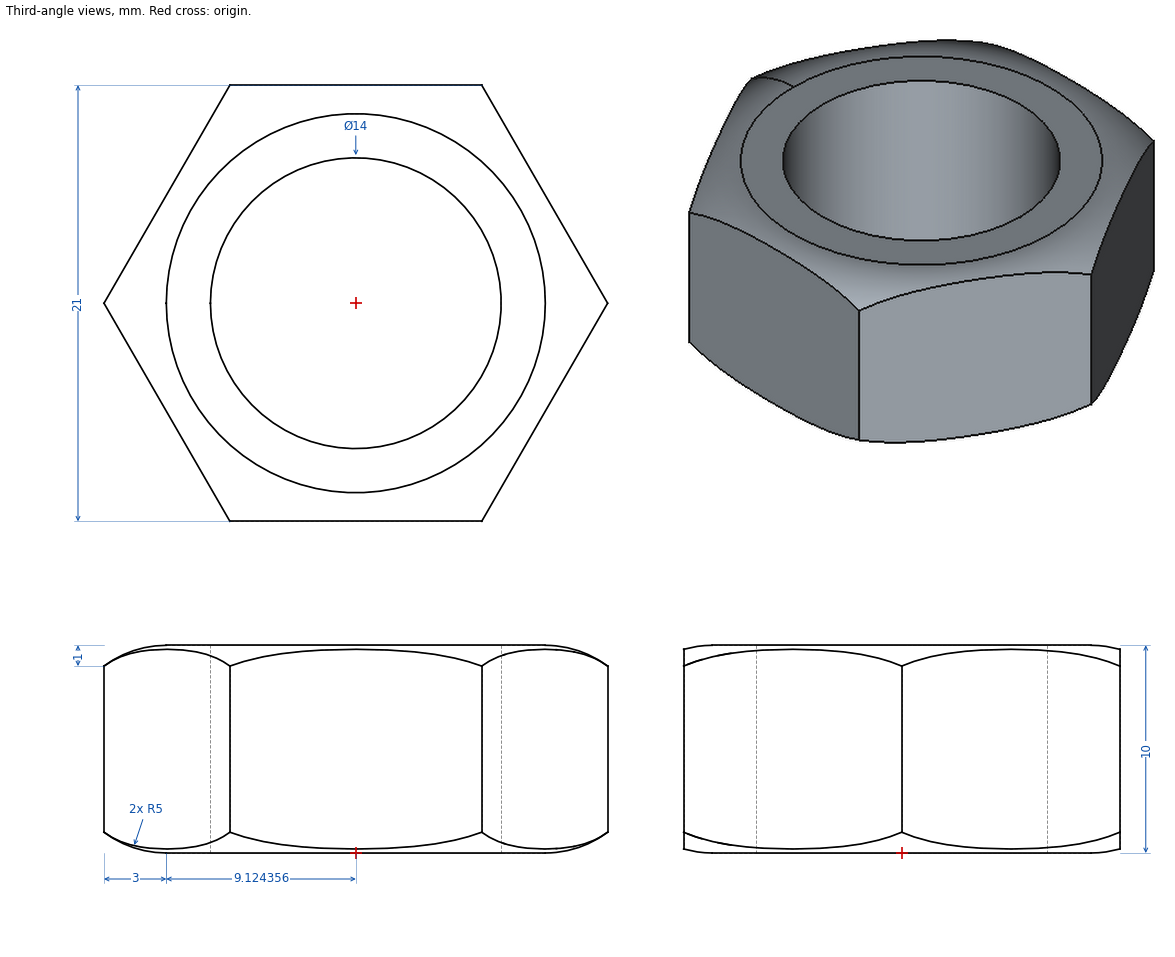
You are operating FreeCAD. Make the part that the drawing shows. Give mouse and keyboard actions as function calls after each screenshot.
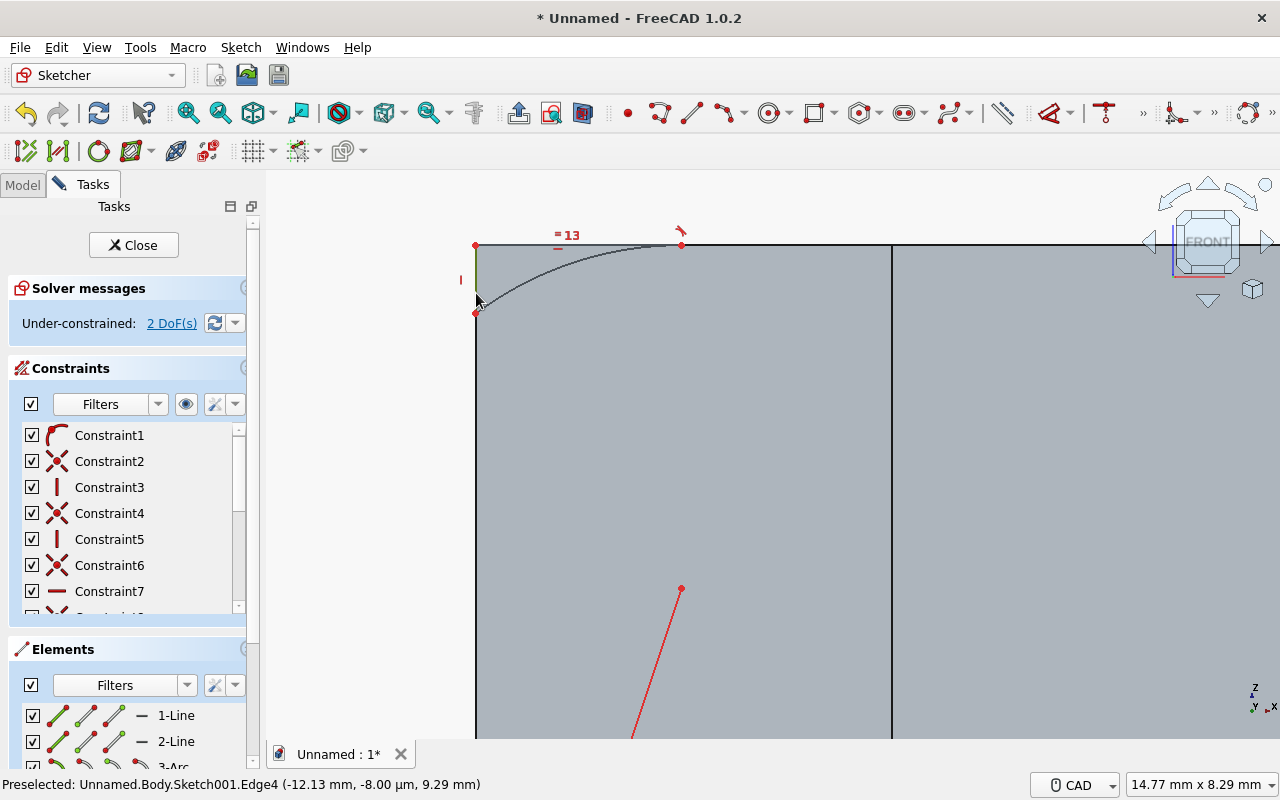
key(i)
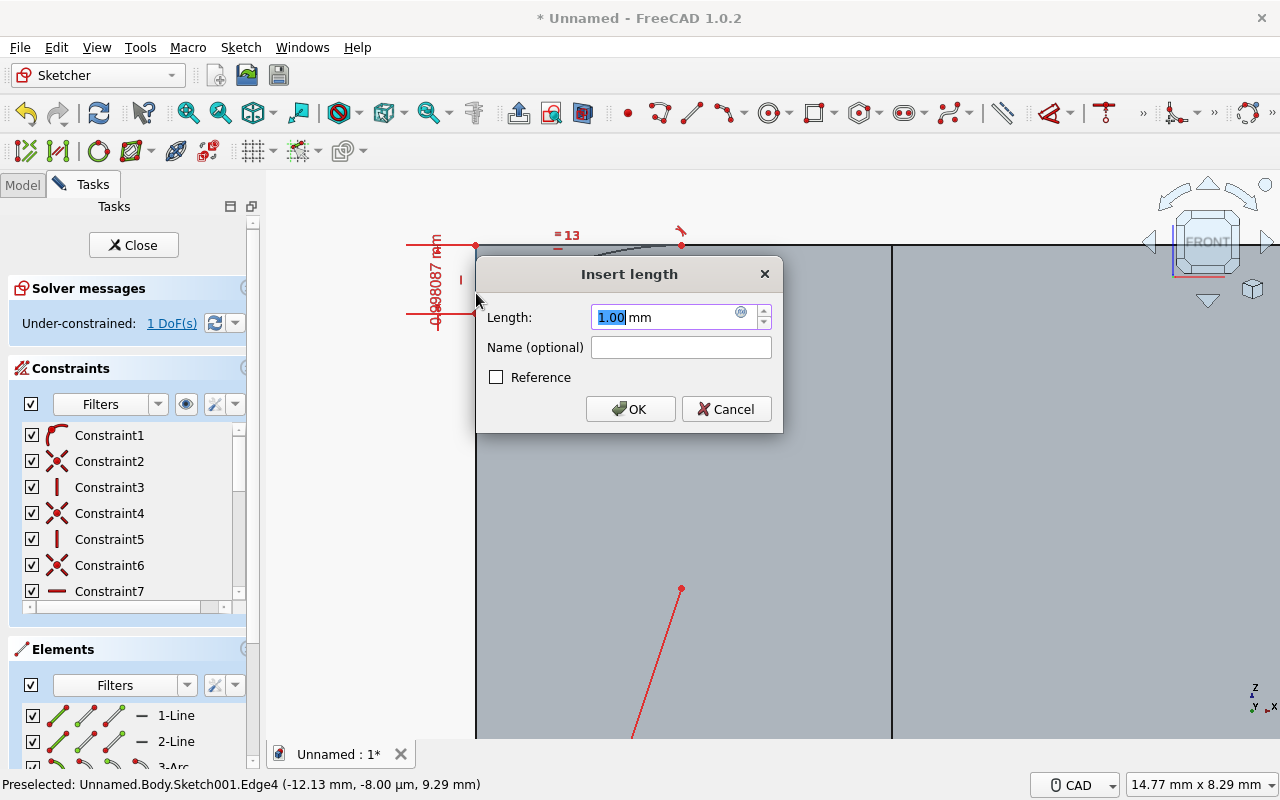
text(1)
key(Return)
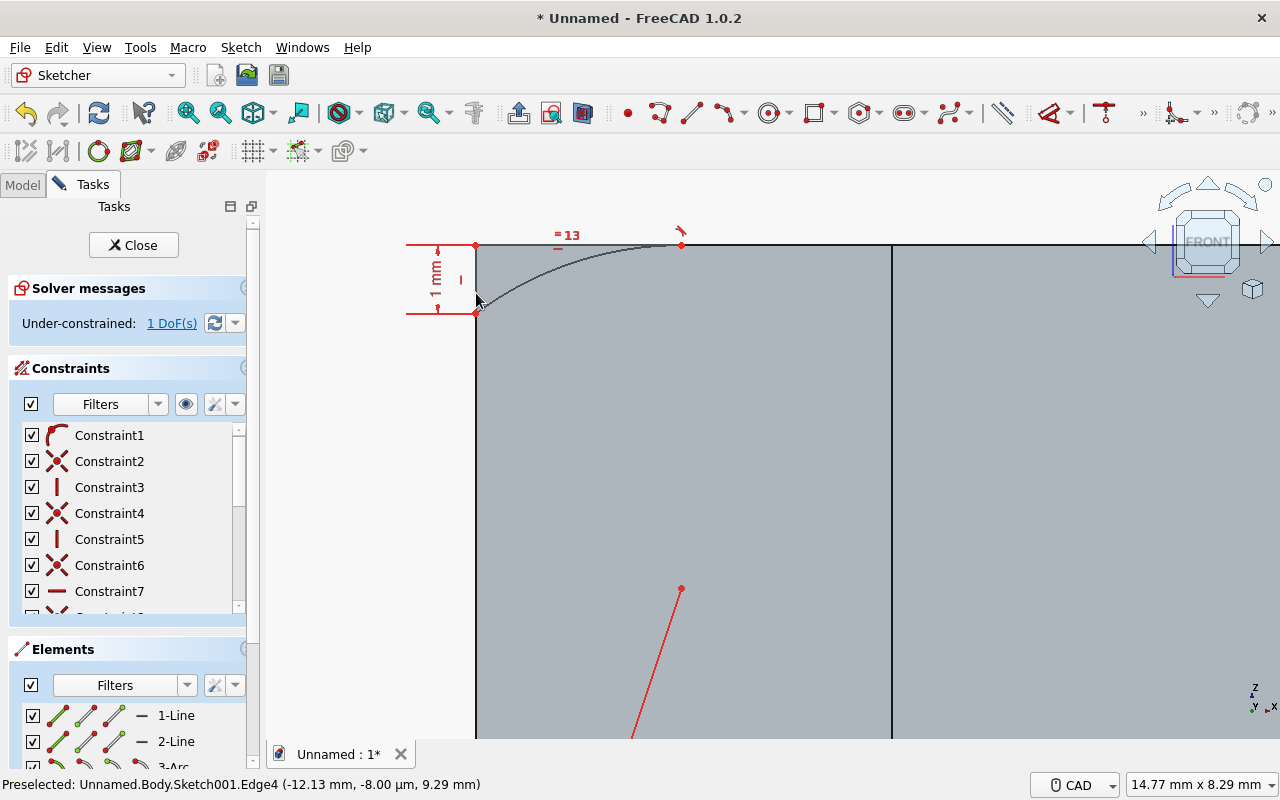
scroll(476, 292, down, 3)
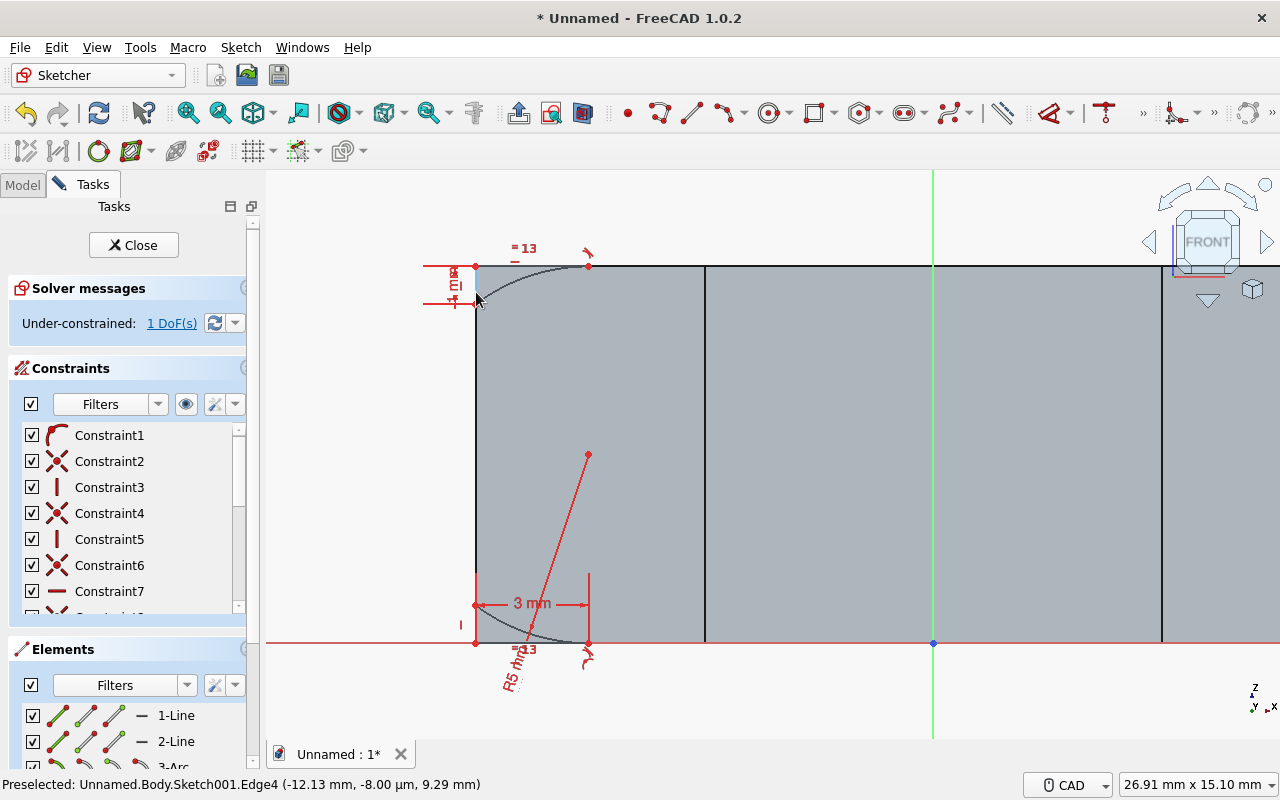
click(589, 643)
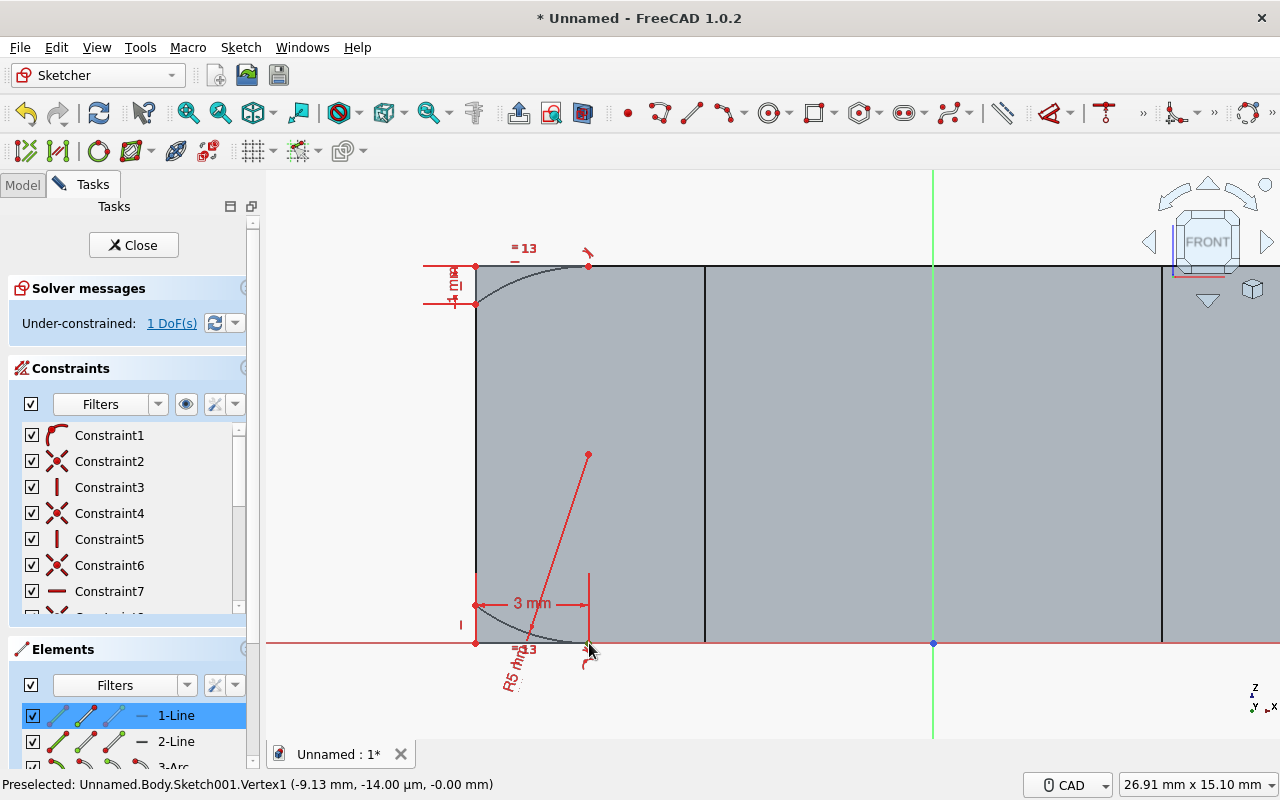
key(l)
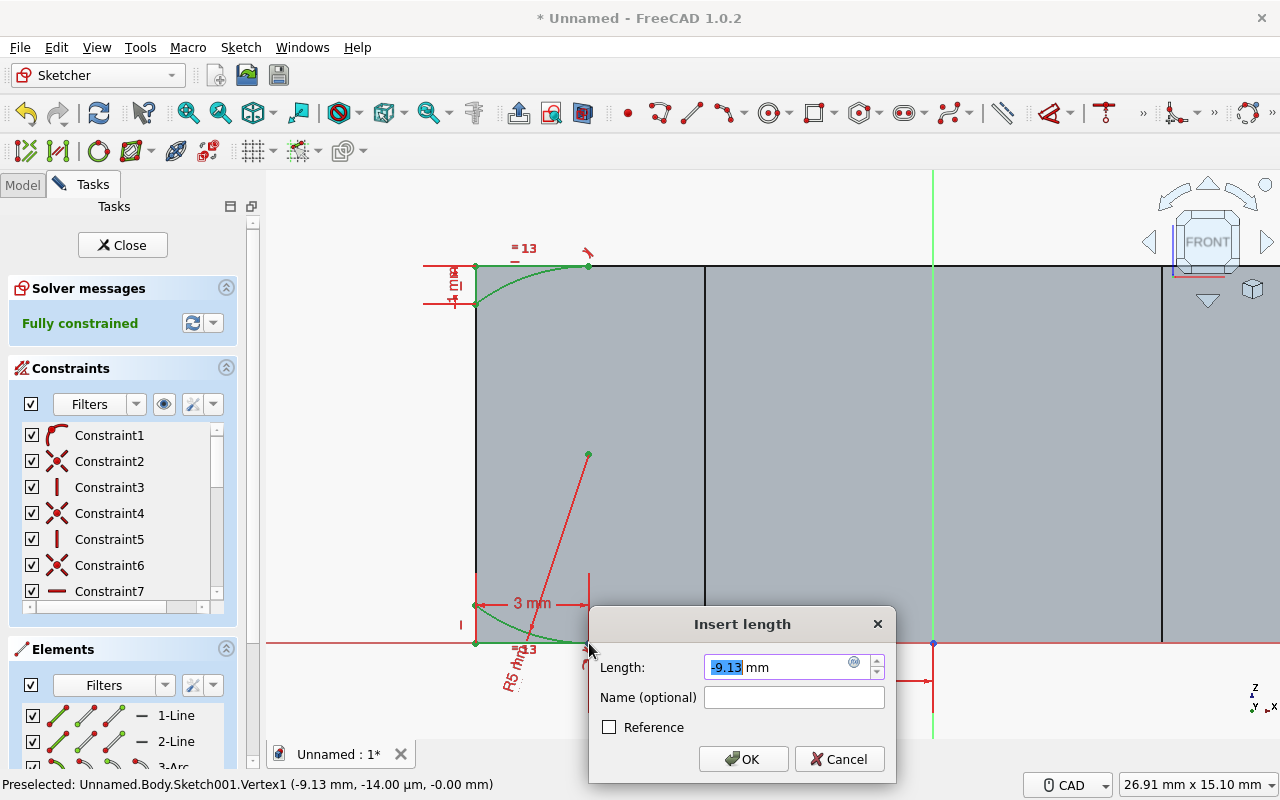
text(-9.124356)
key(Return)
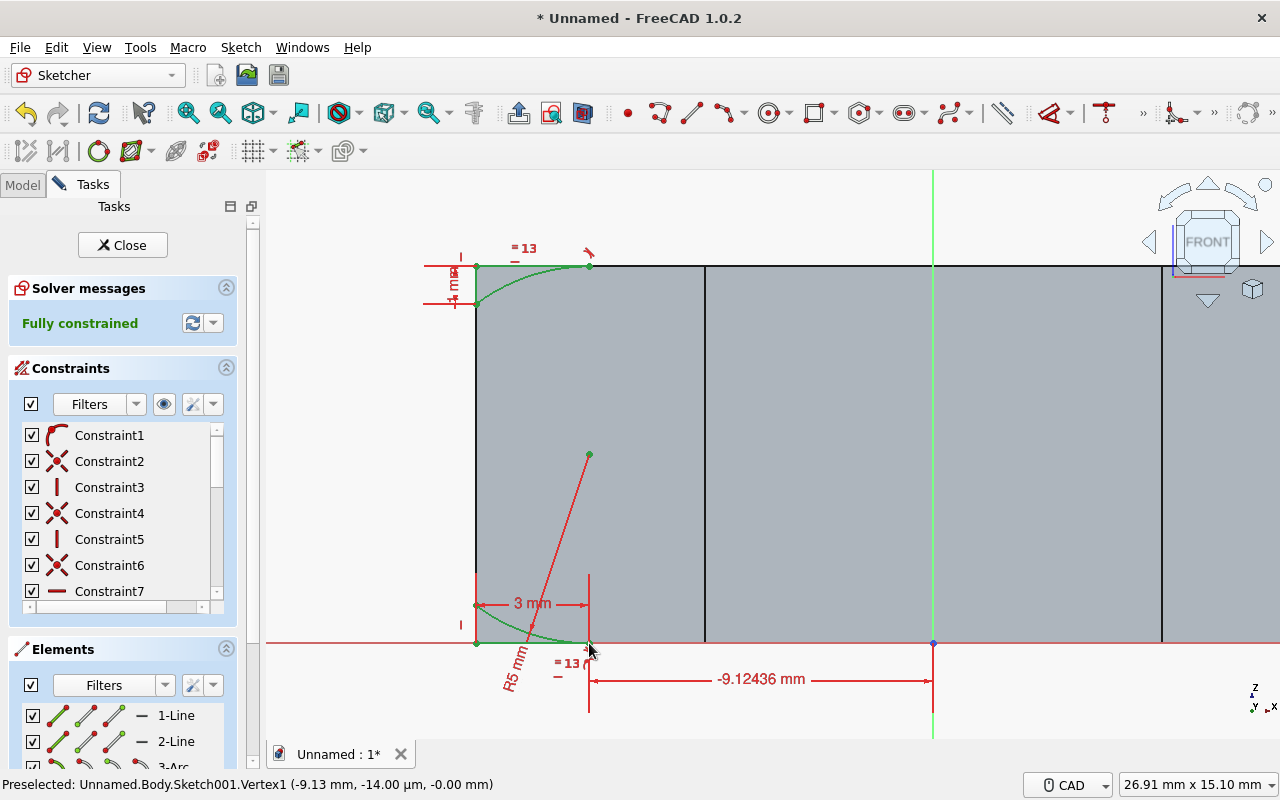
click(123, 245)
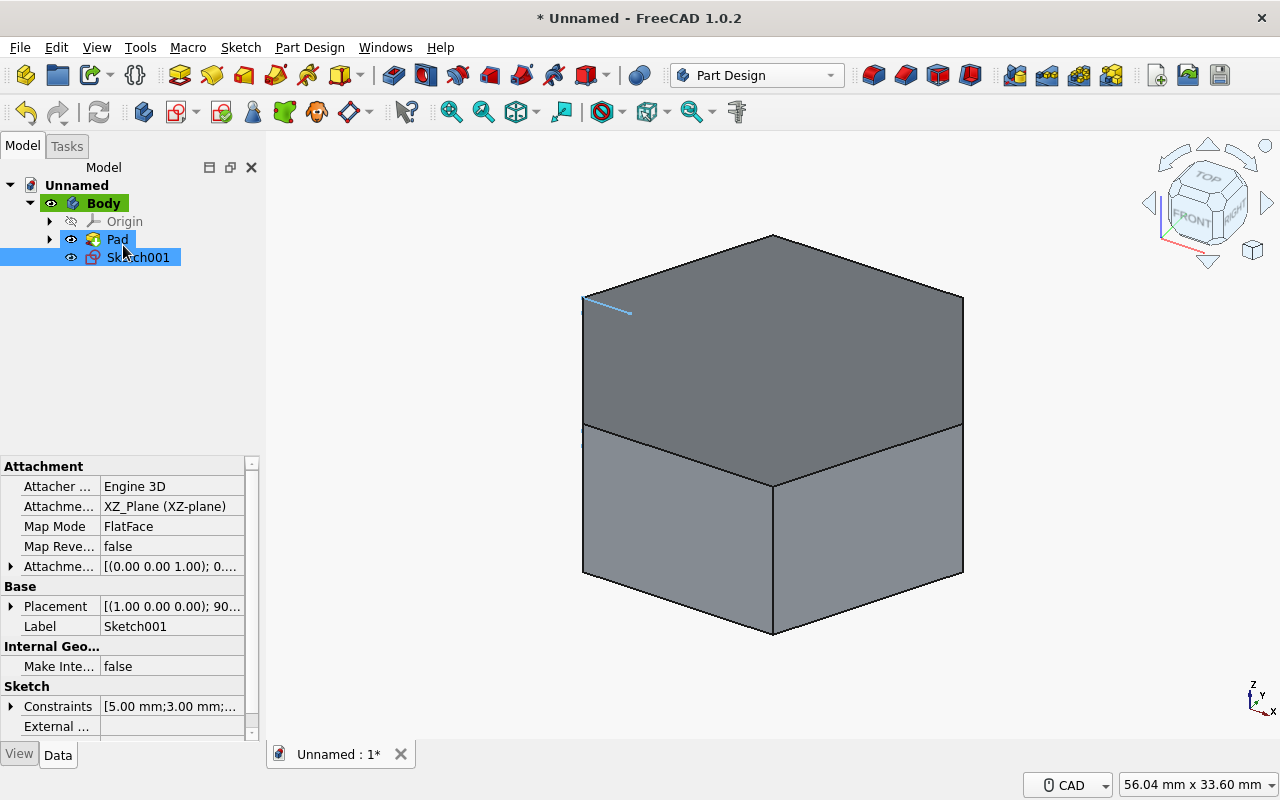
click(458, 76)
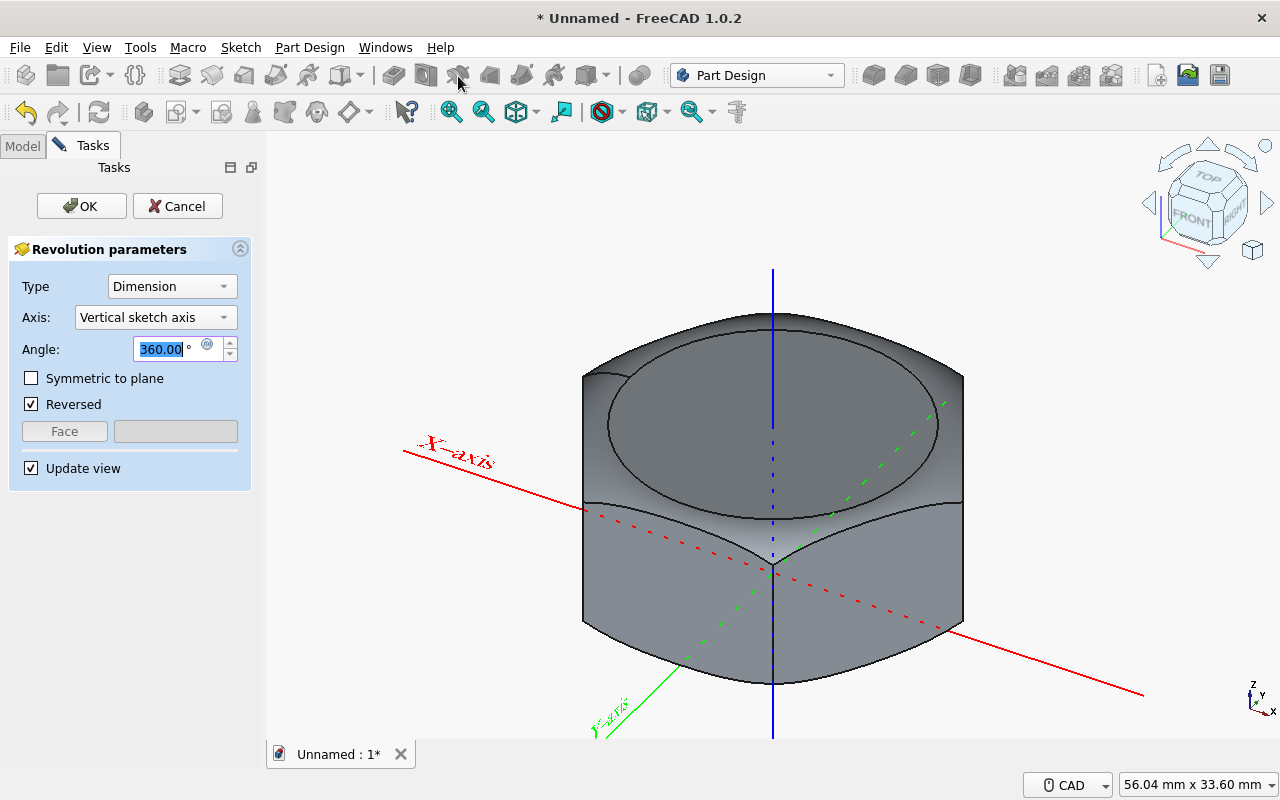
click(82, 206)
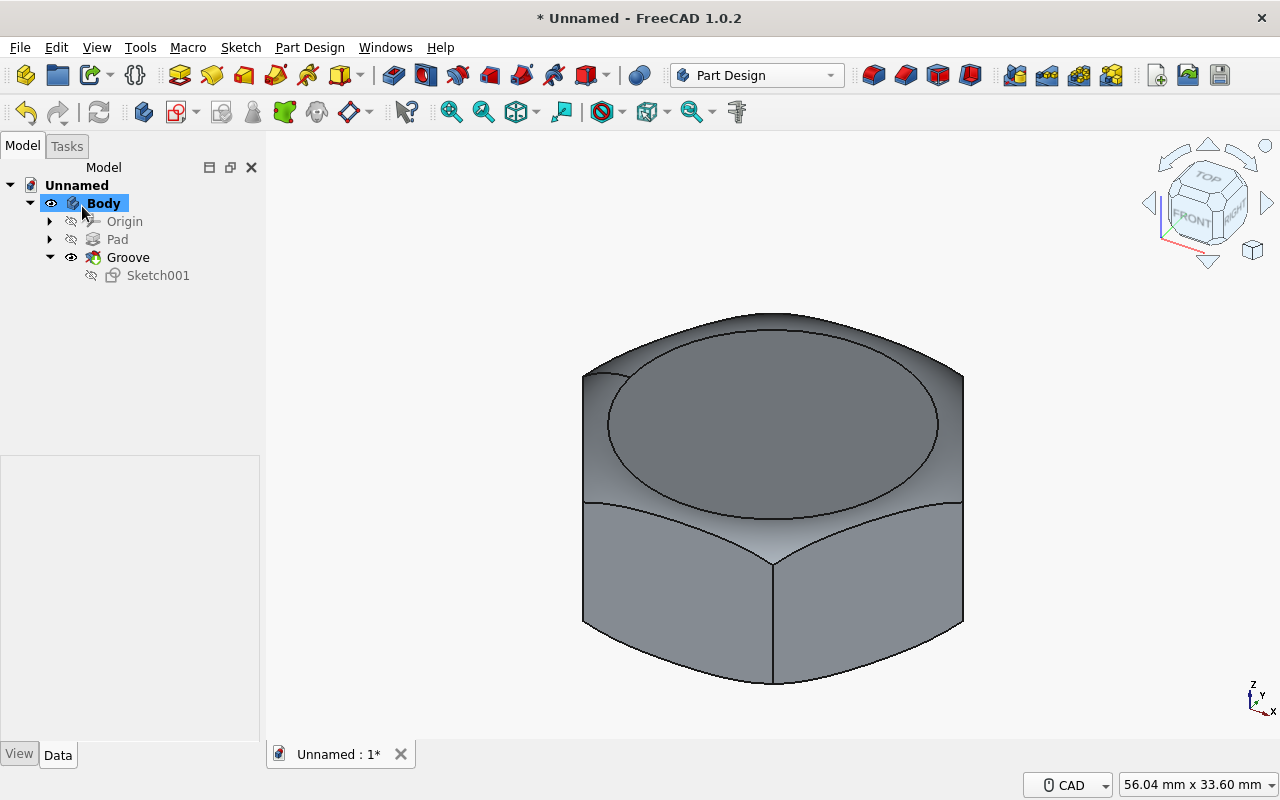
click(176, 112)